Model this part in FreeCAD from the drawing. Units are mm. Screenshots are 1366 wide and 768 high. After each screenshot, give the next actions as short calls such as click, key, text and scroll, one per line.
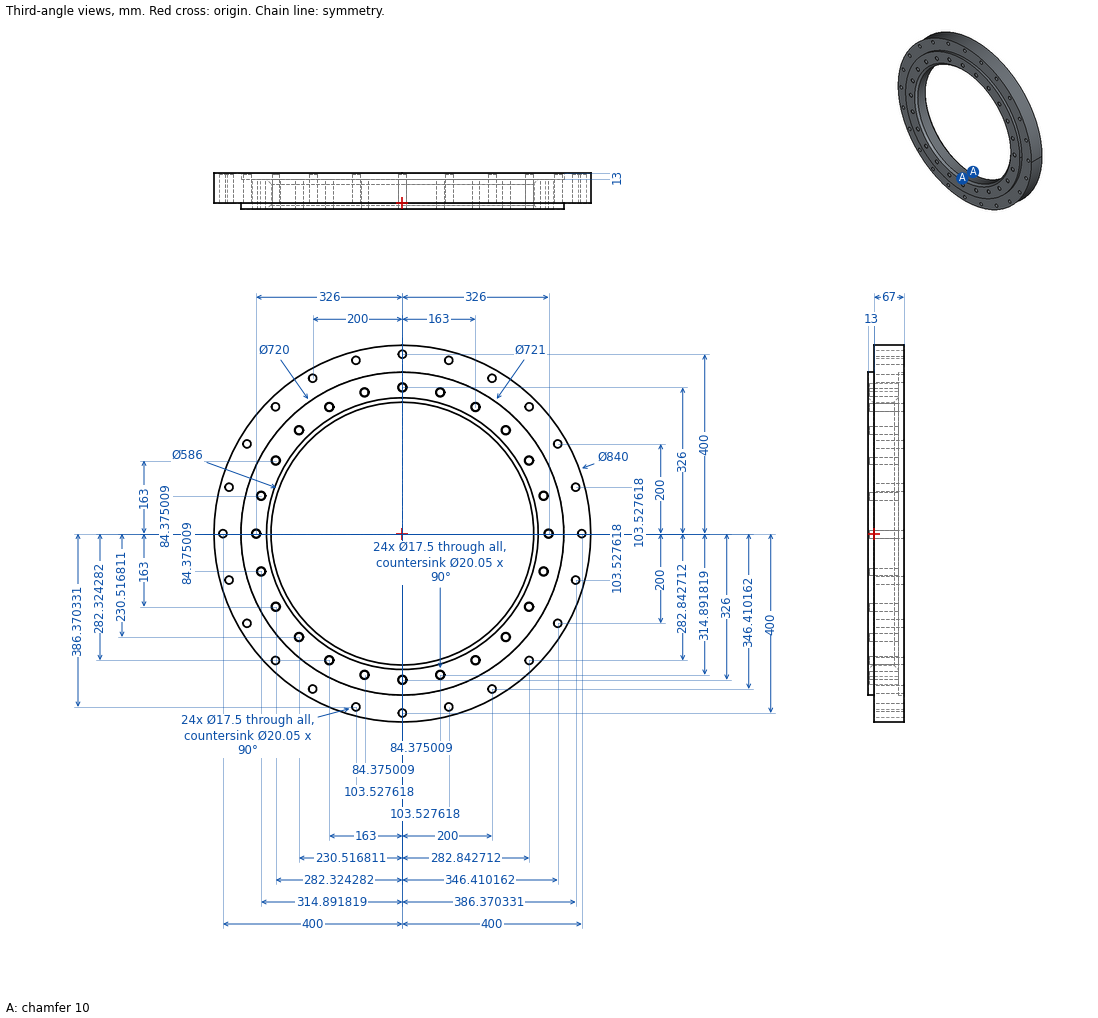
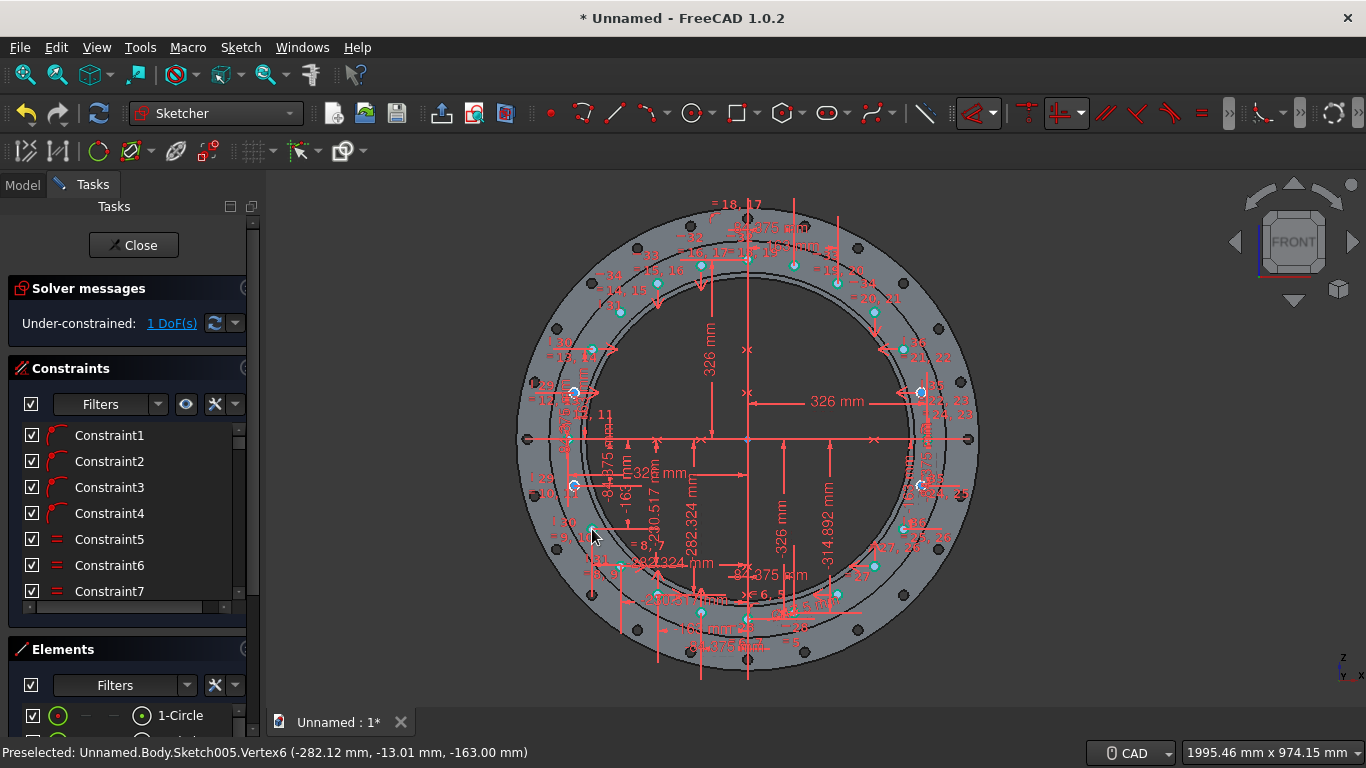
click(574, 486)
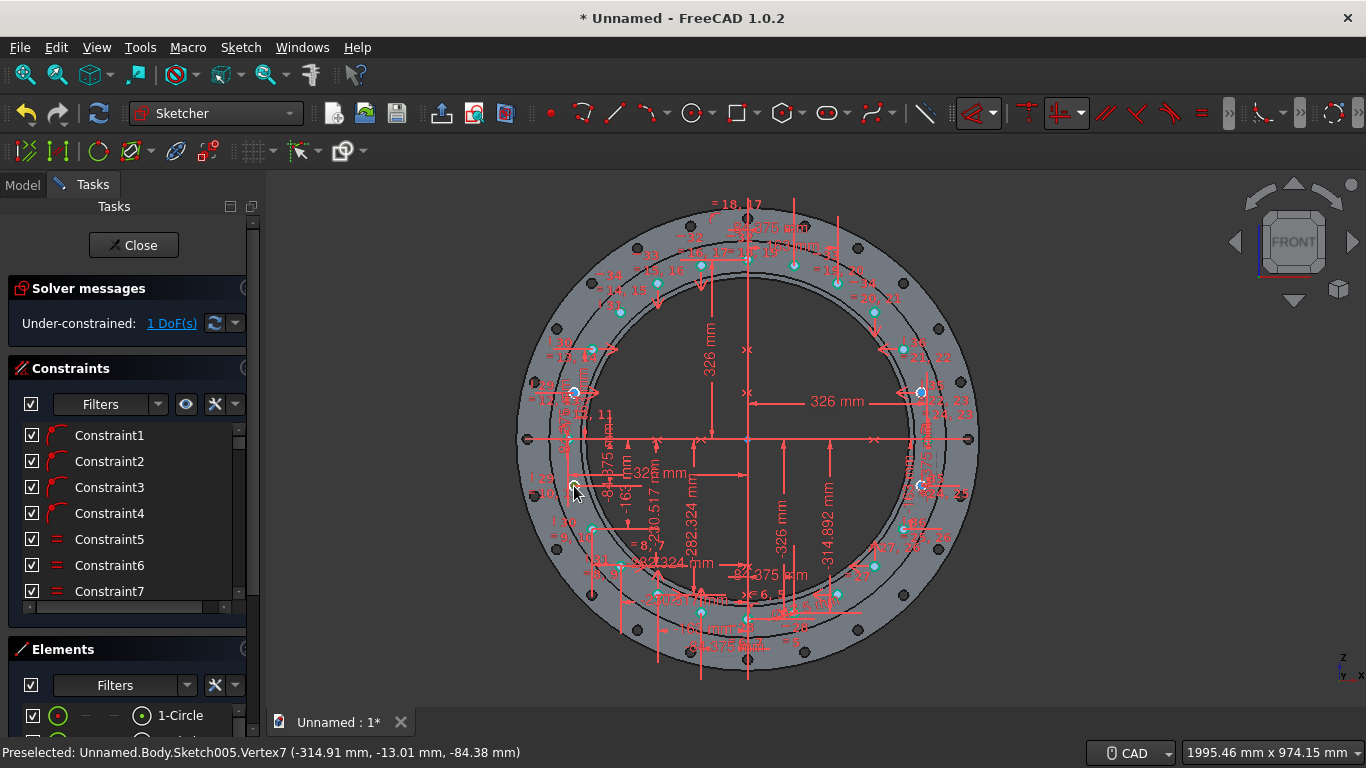
click(996, 114)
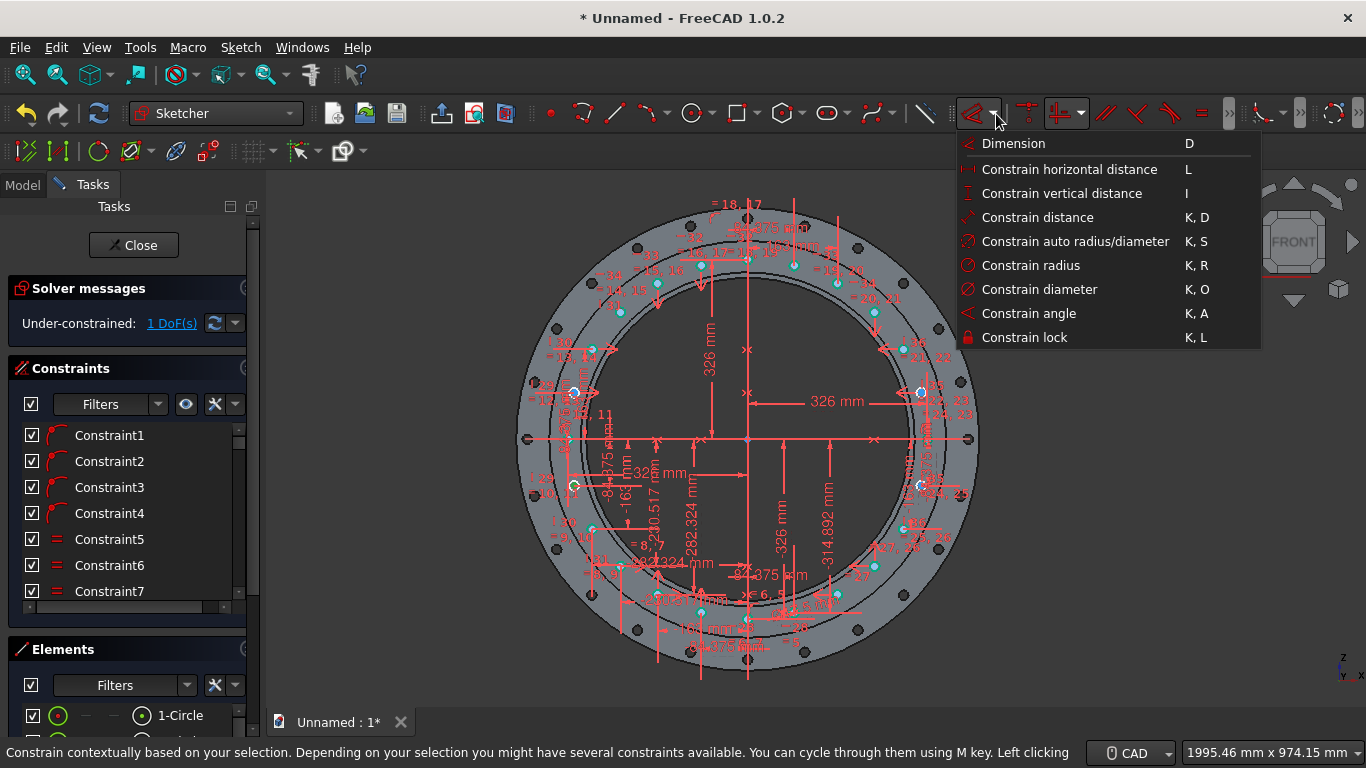
click(1109, 169)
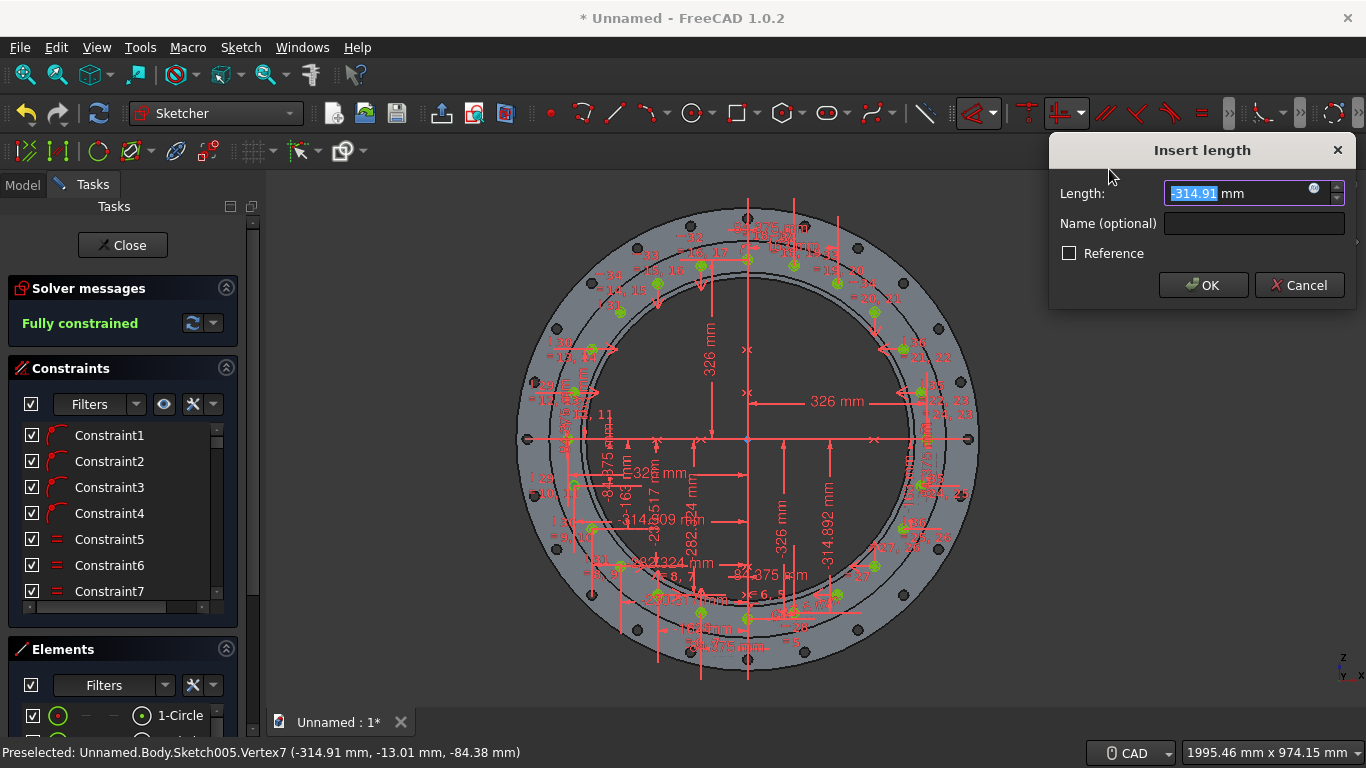
text(-314.891819)
key(Return)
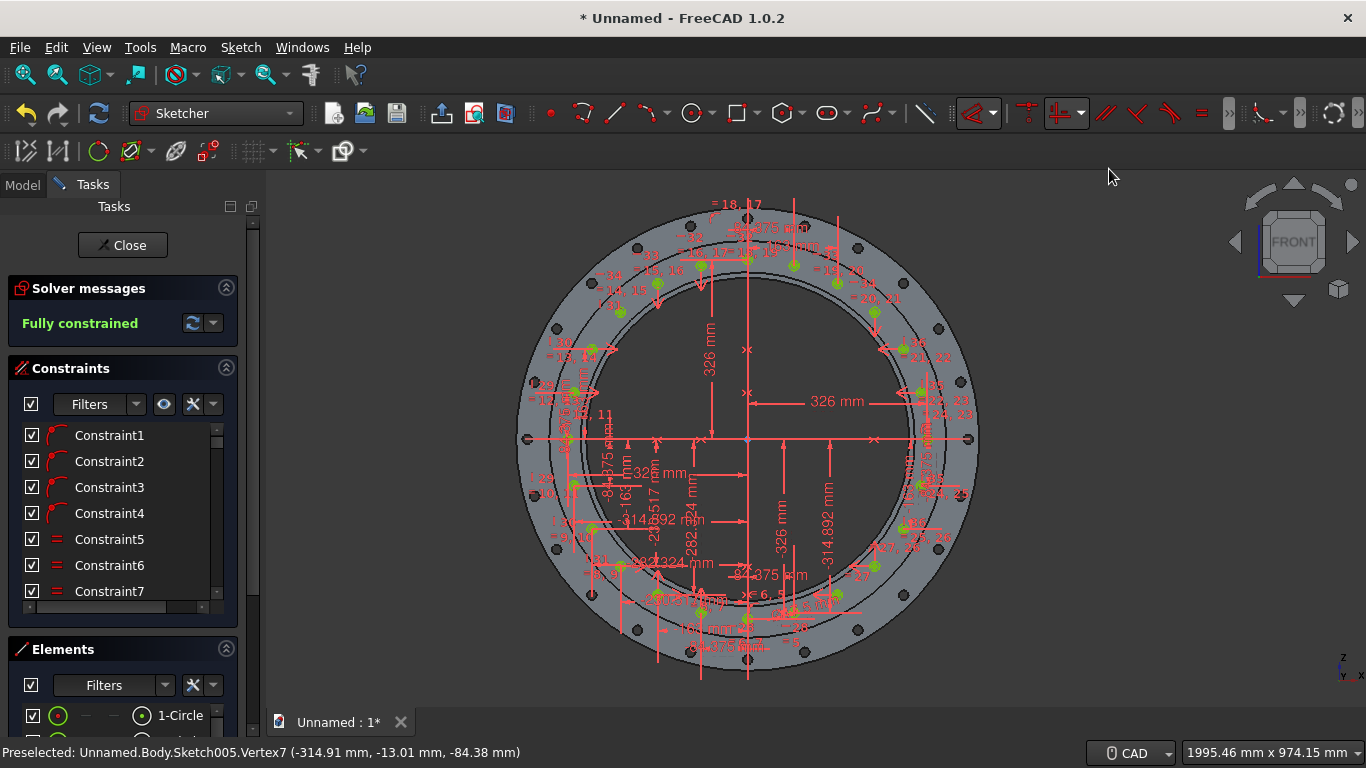
click(123, 245)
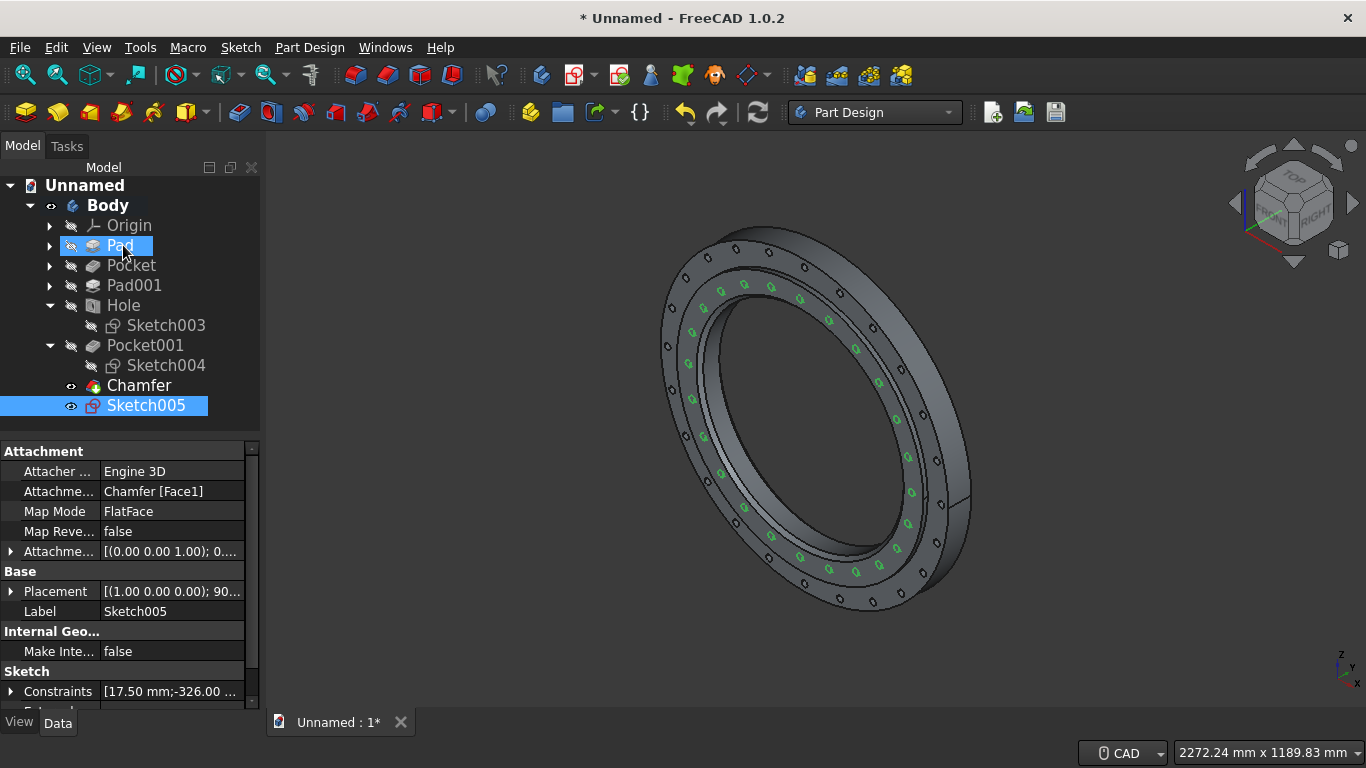
click(272, 112)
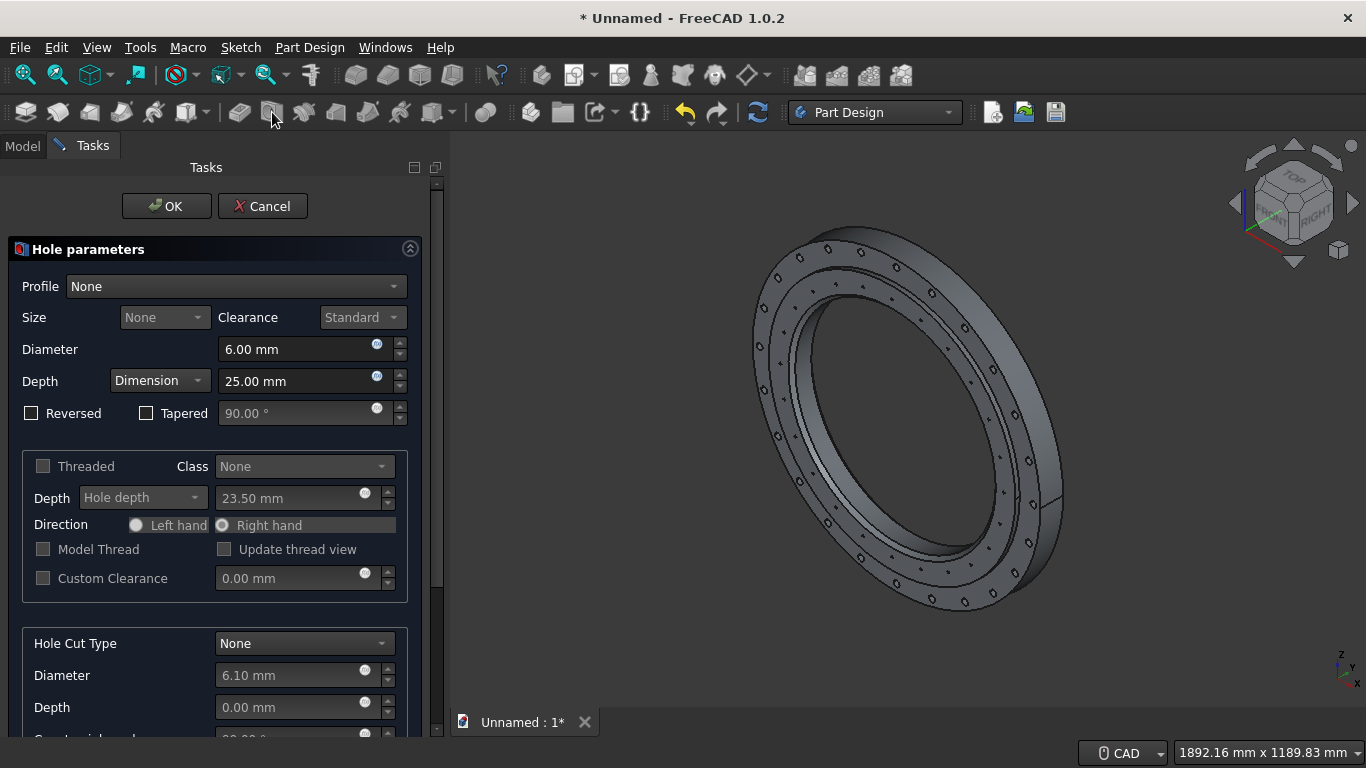
triple_click(305, 349)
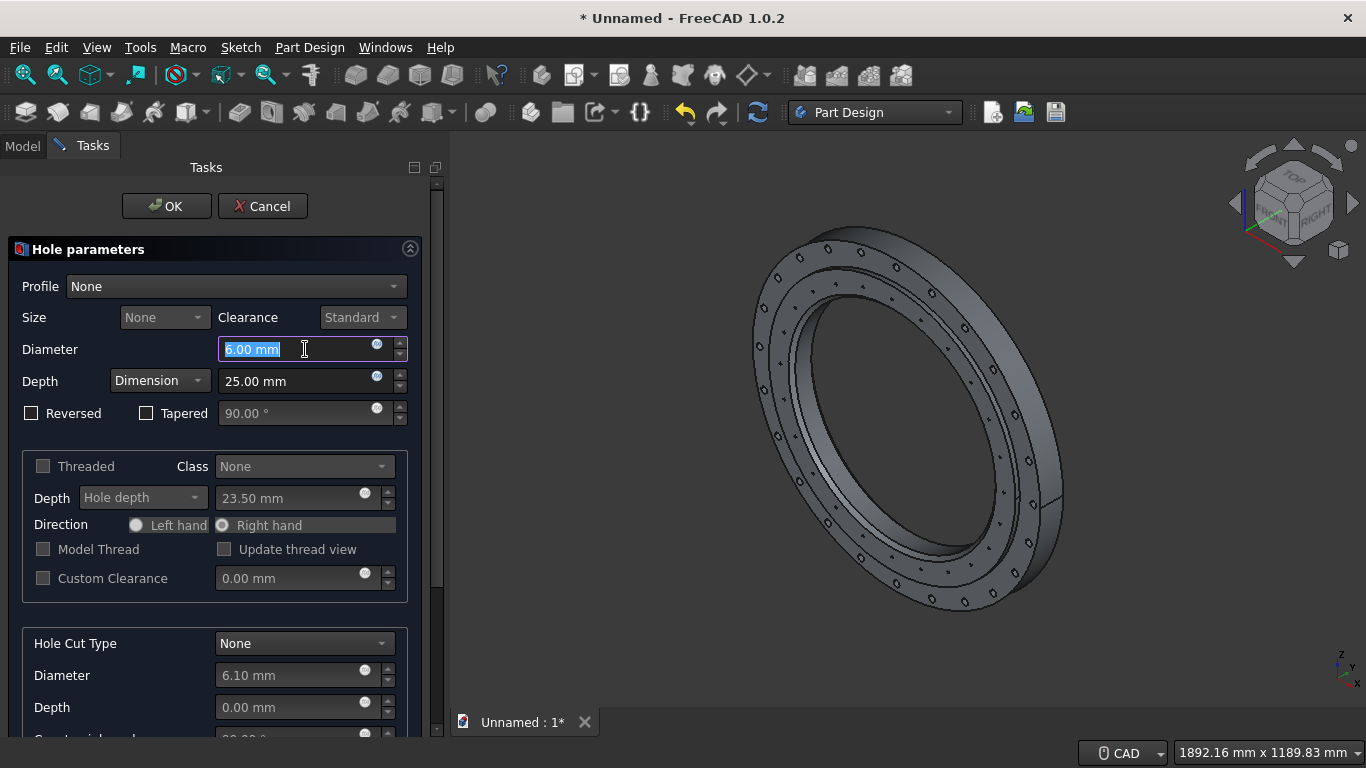
text(17.5)
key(Tab)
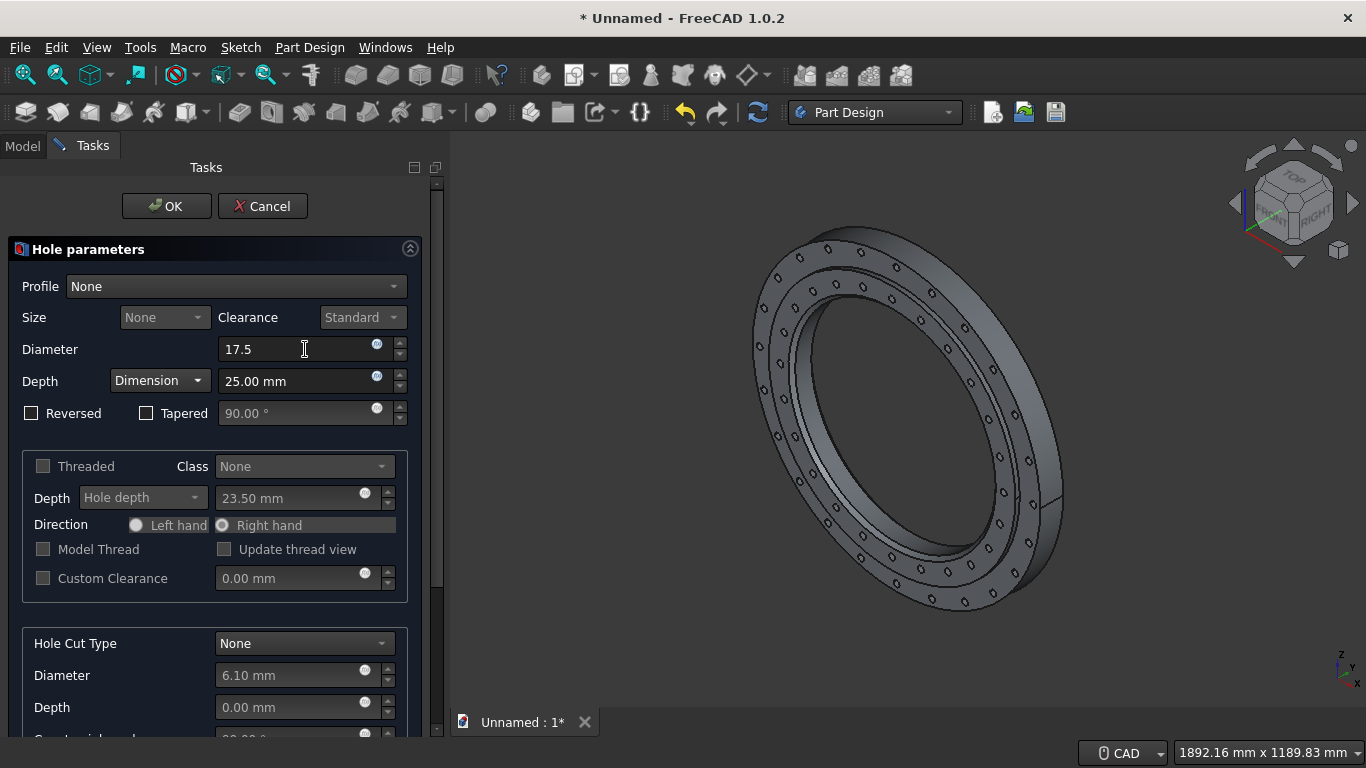
click(161, 380)